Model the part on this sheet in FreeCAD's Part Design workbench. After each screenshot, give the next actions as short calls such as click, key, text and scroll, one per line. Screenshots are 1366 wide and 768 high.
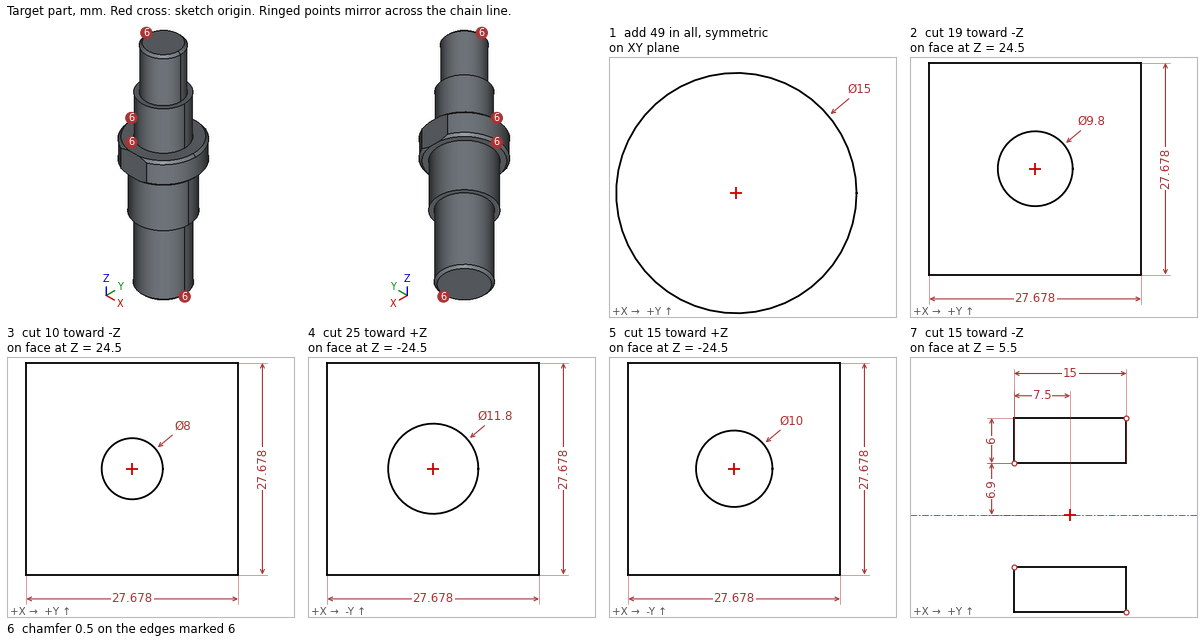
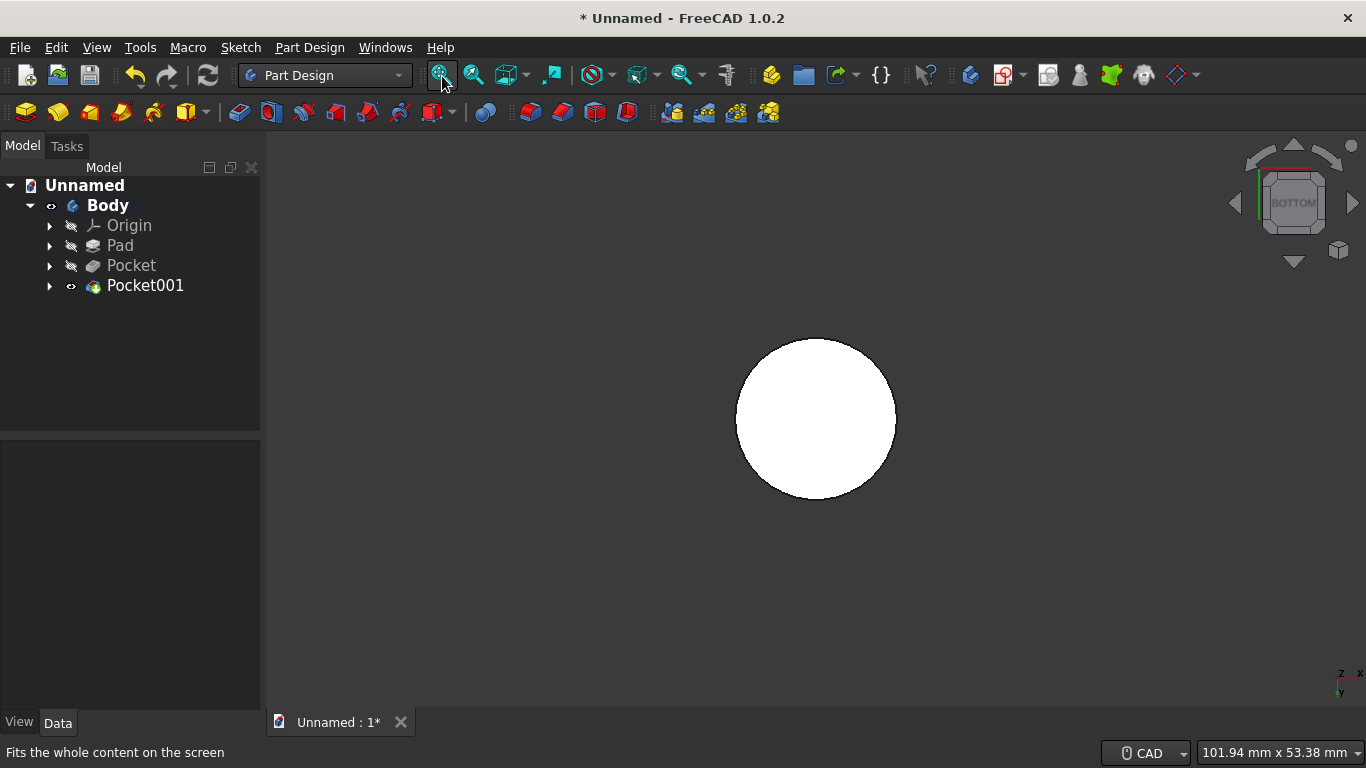
click(816, 418)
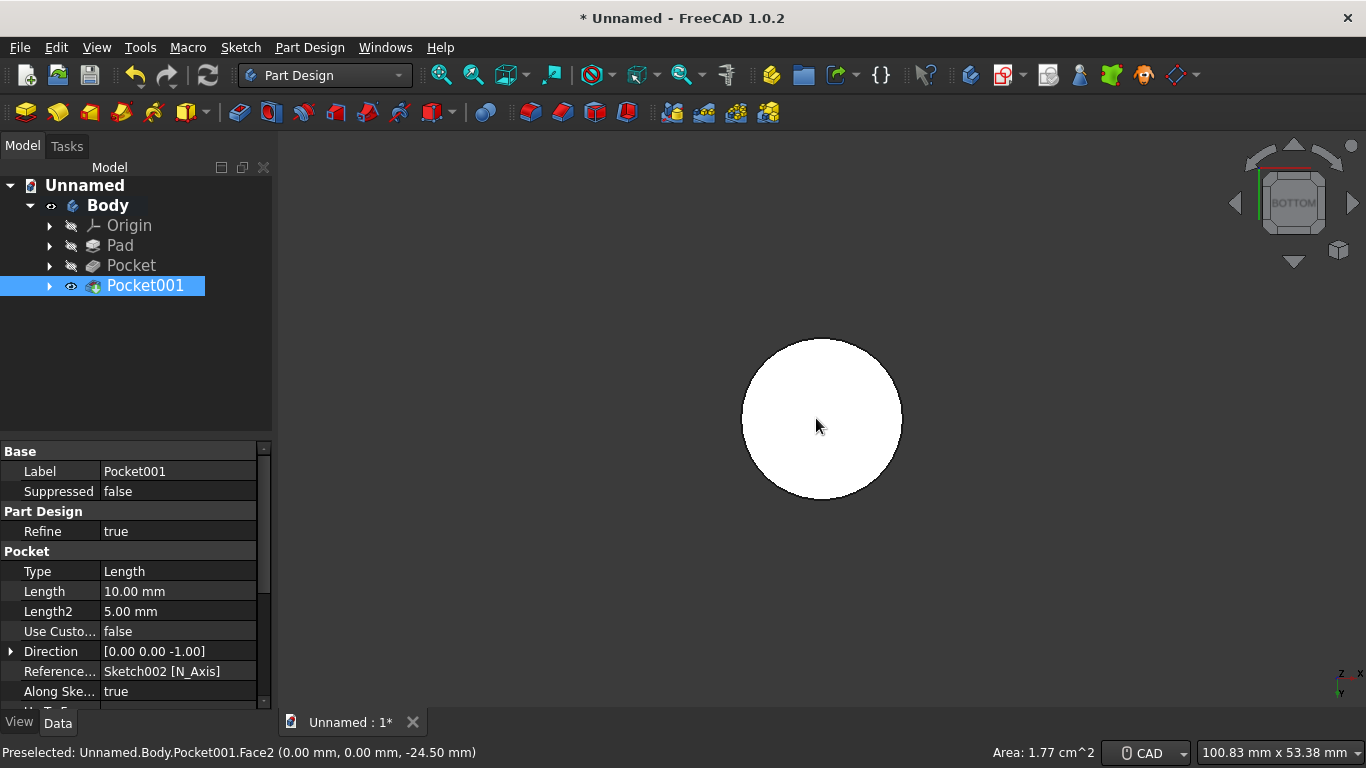
click(1004, 76)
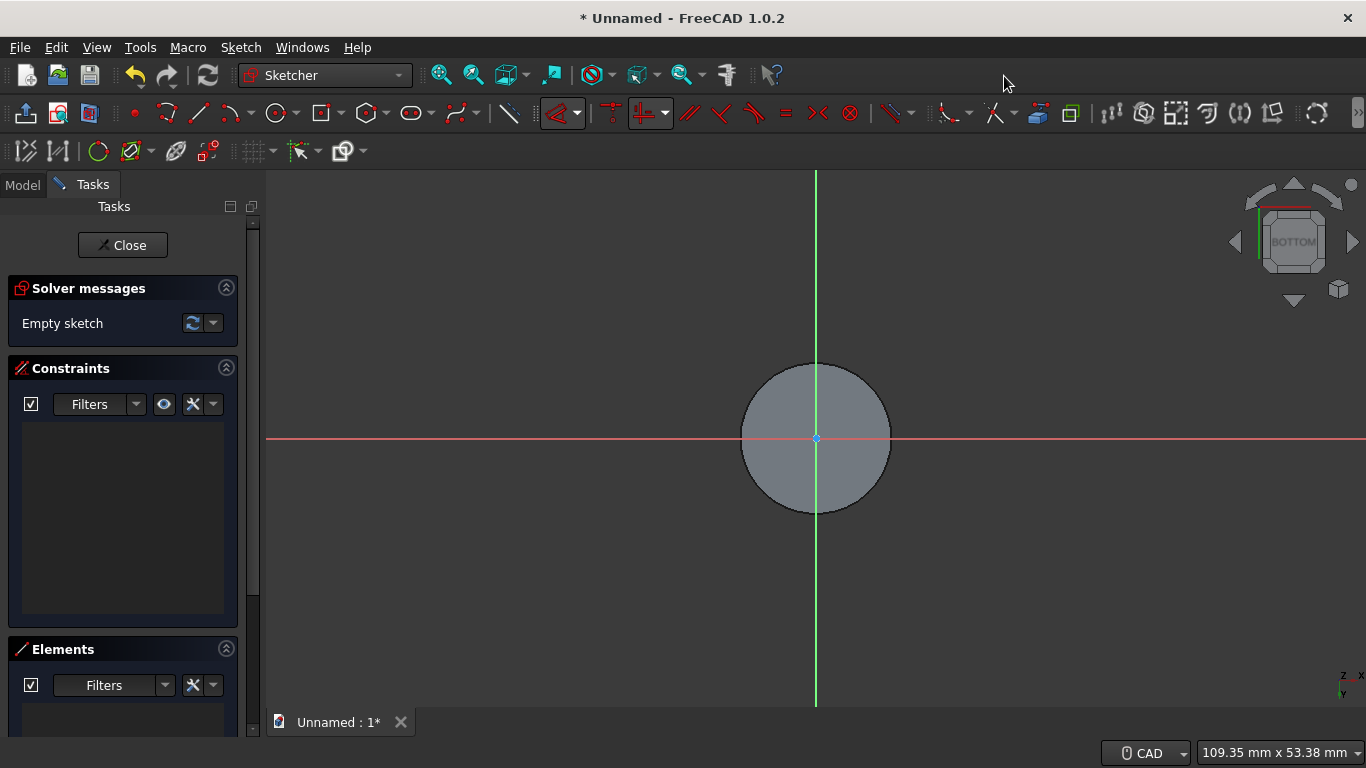
click(322, 114)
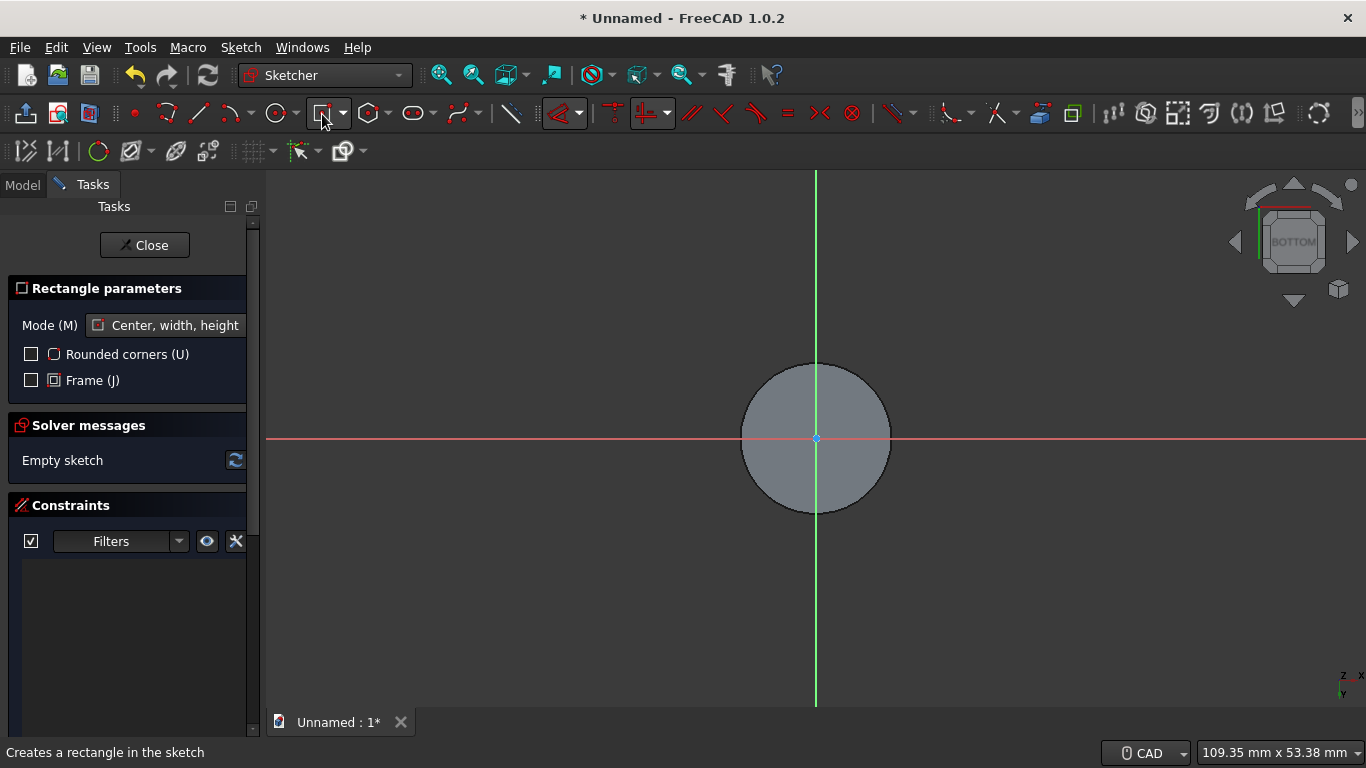
click(816, 438)
click(955, 299)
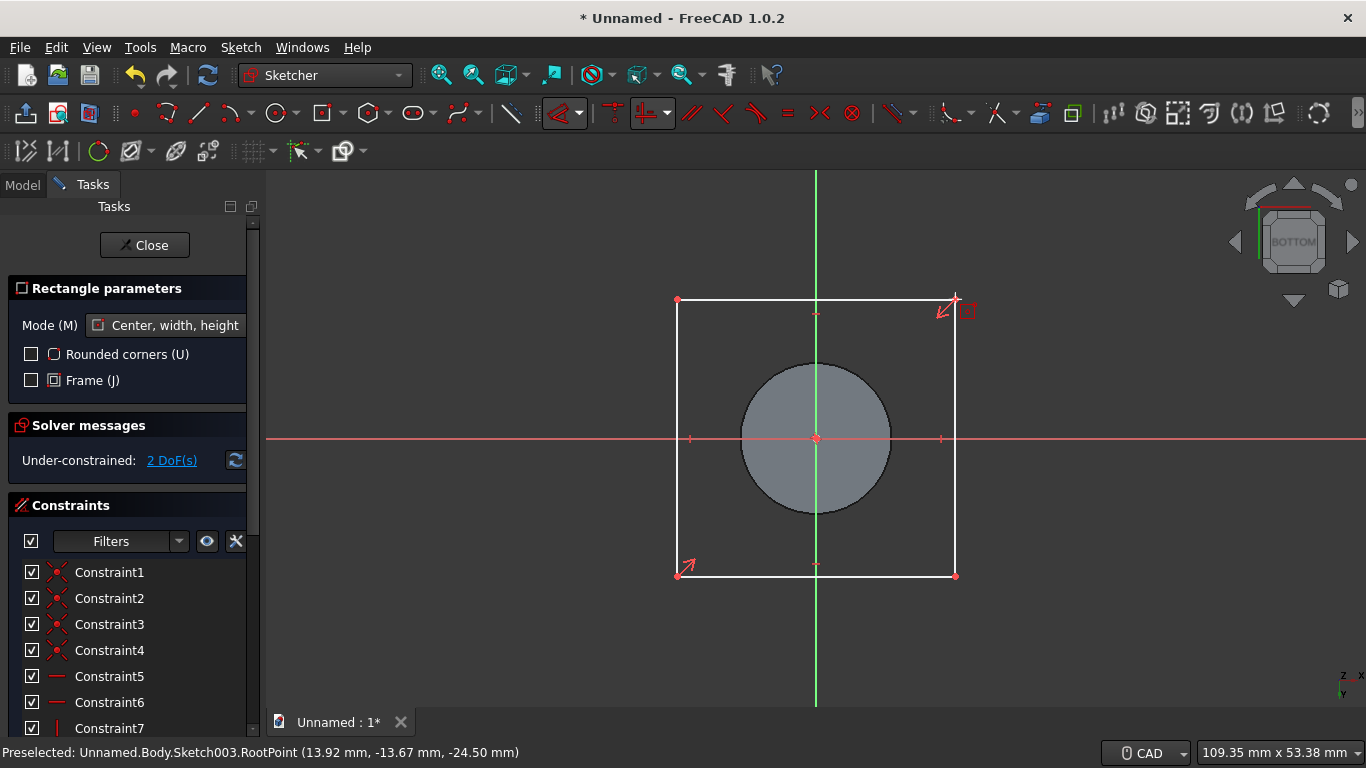
click(276, 114)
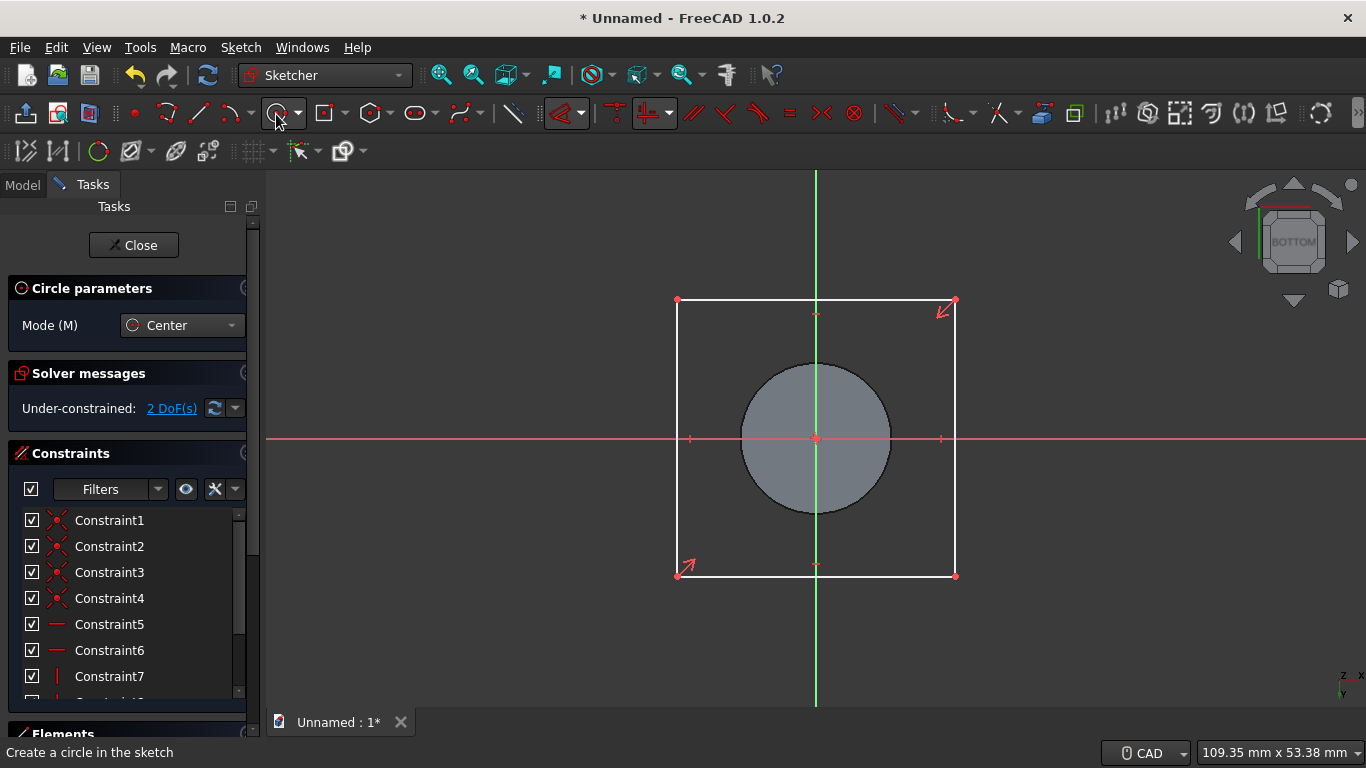
click(816, 438)
click(858, 397)
key(Escape)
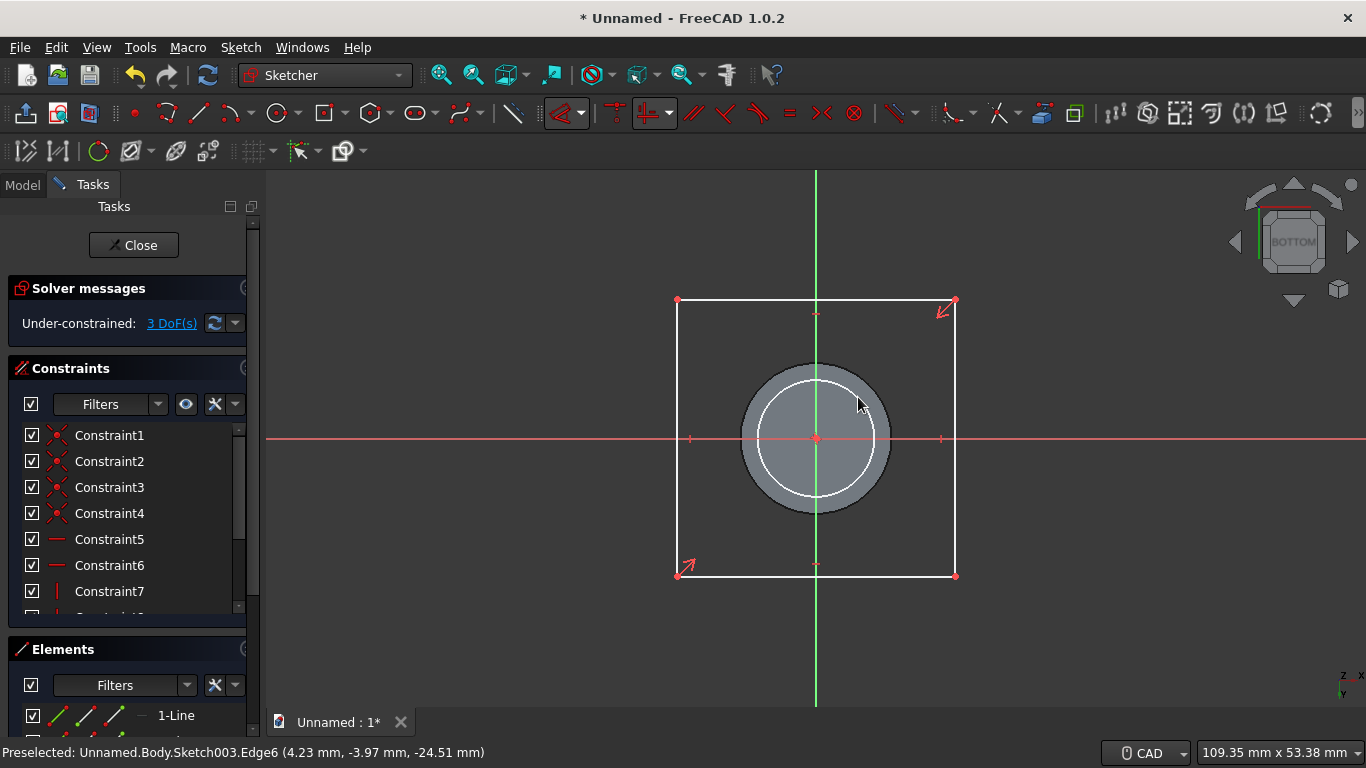
click(857, 397)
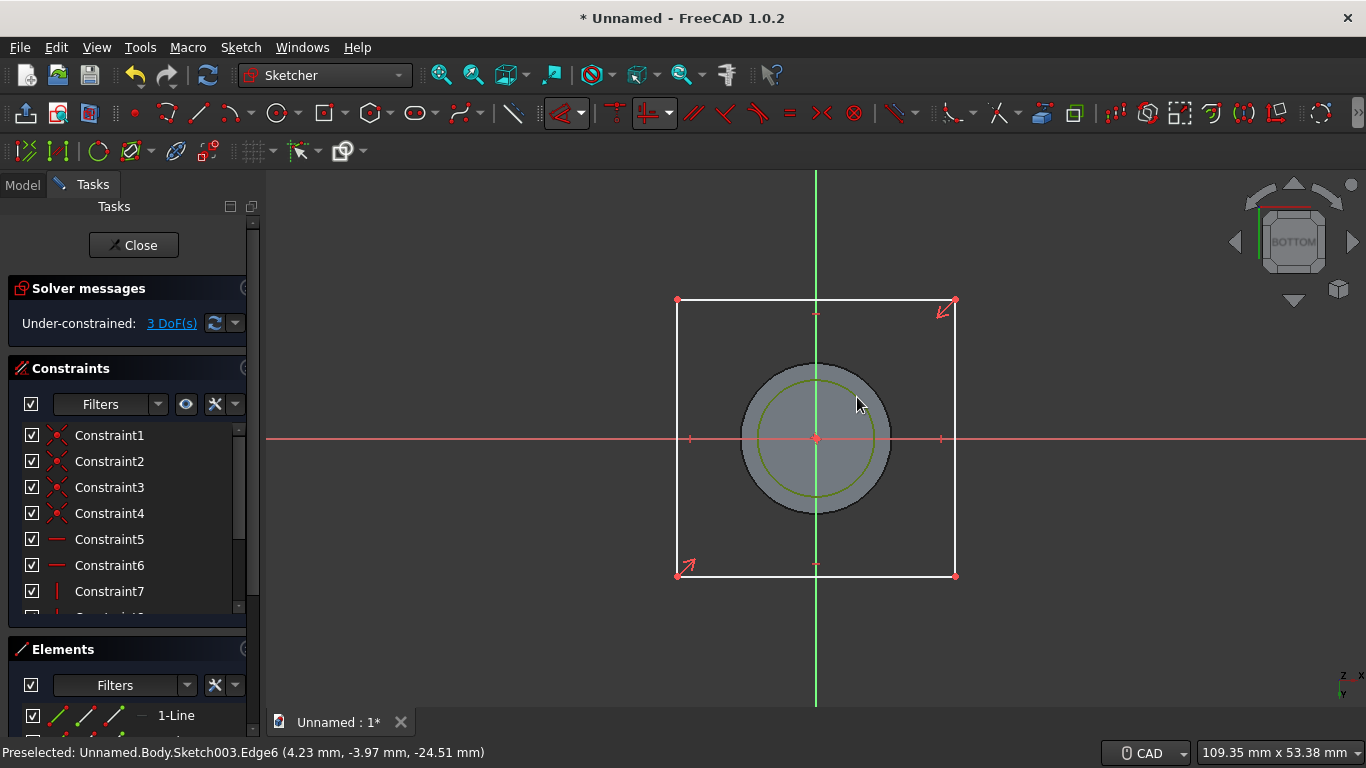
click(584, 114)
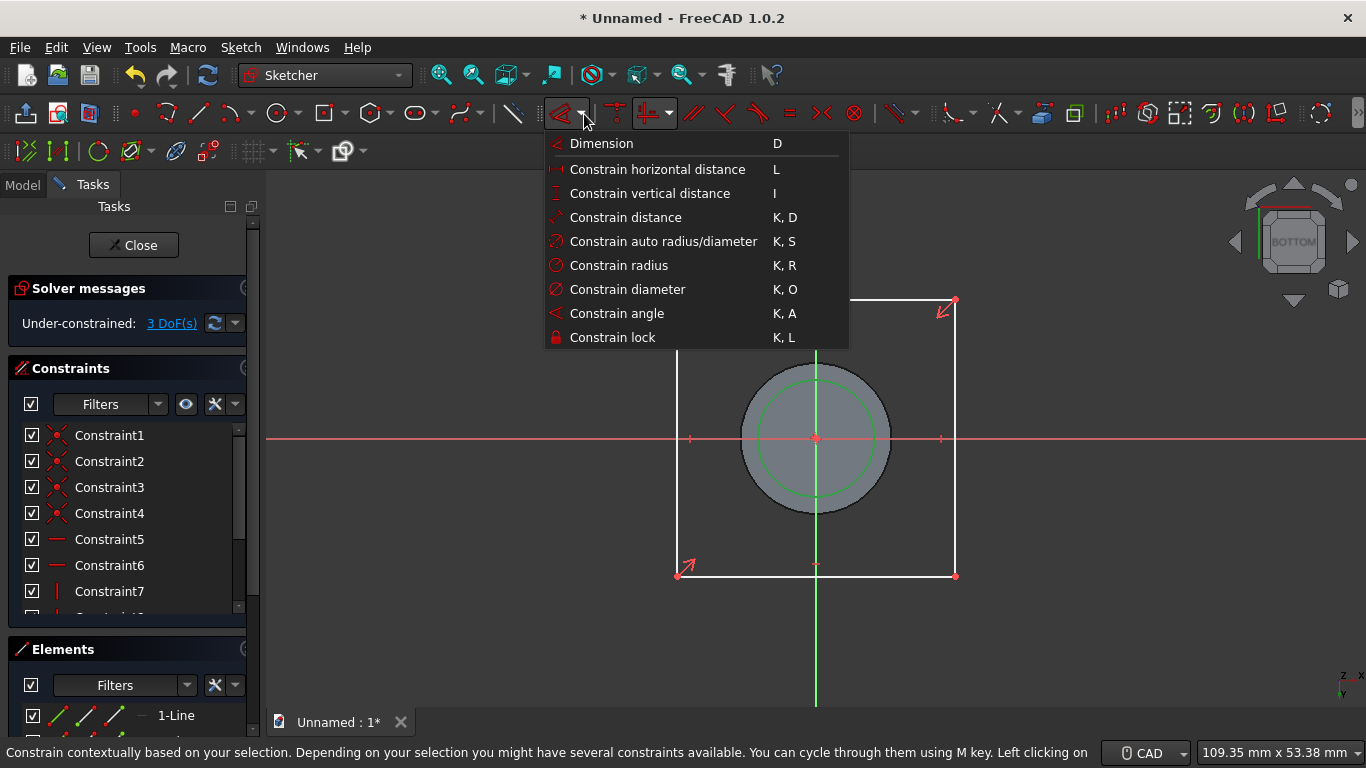
click(697, 289)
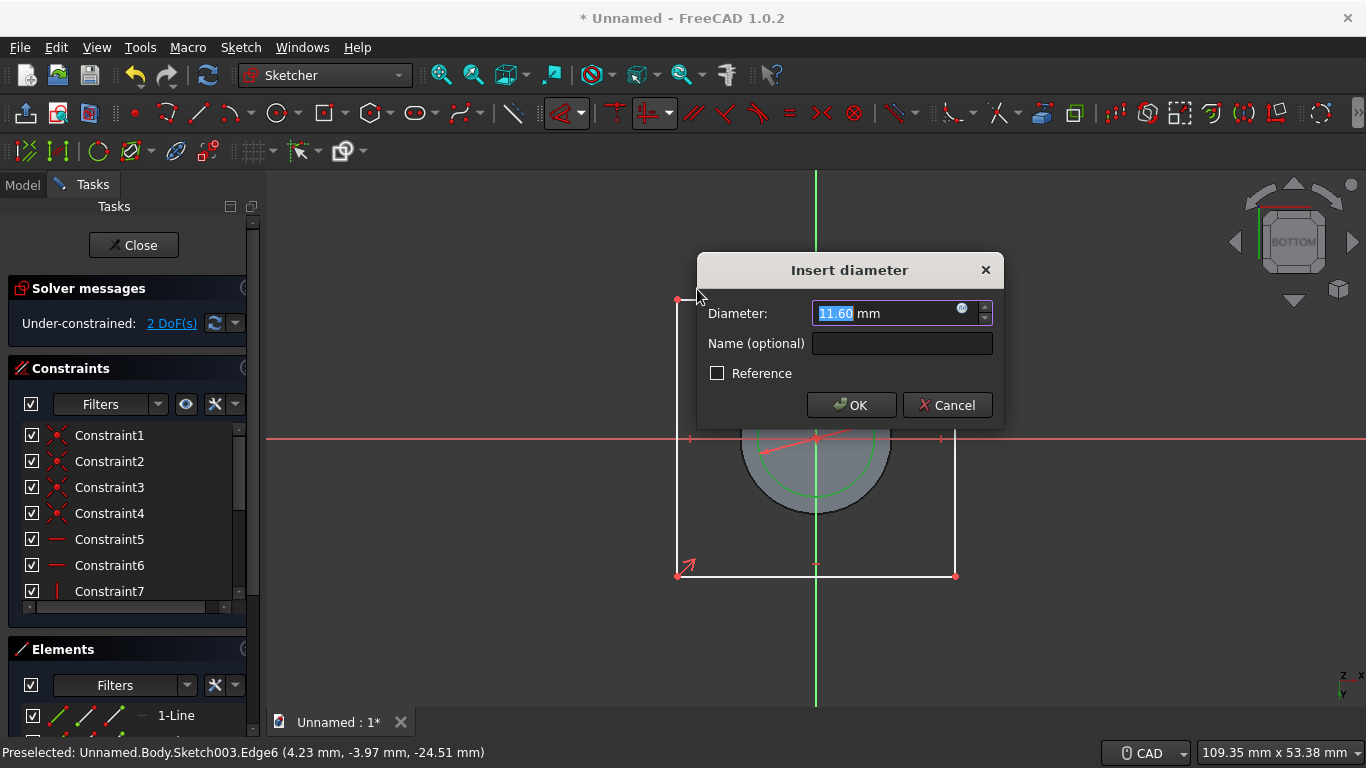
text(11.8)
key(Return)